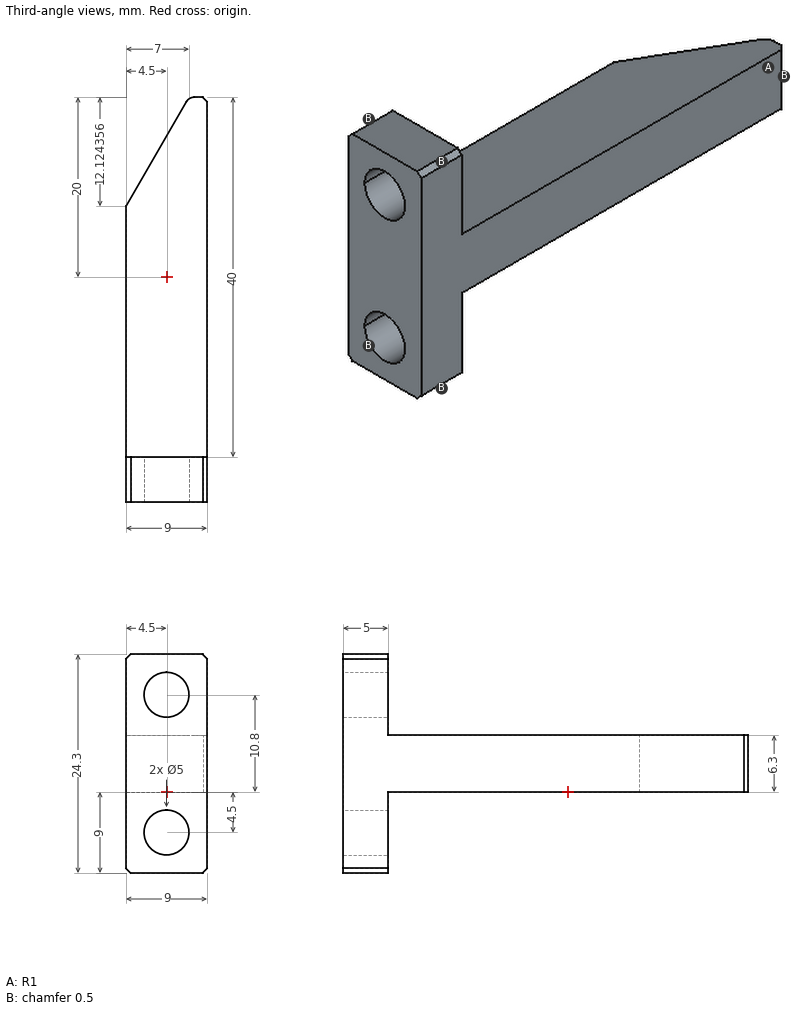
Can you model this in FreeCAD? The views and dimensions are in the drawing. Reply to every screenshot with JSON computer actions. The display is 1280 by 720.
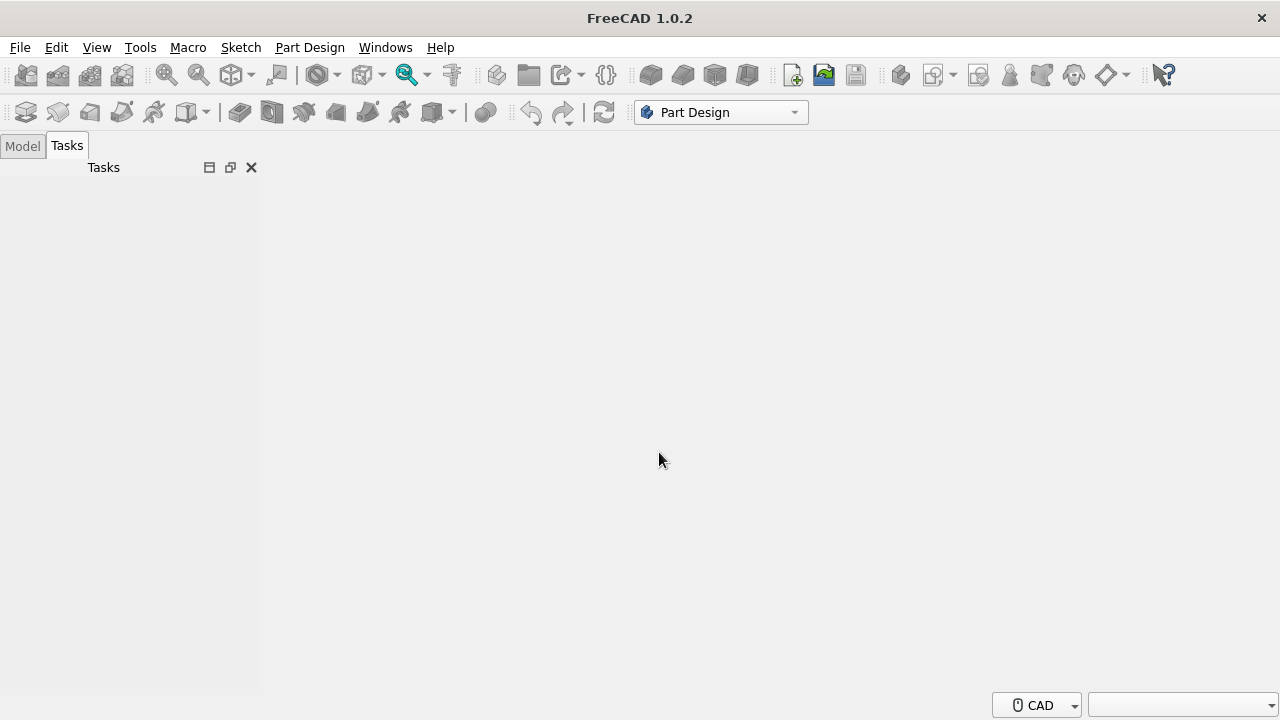
{"action": "left_click", "coordinate": [792, 76]}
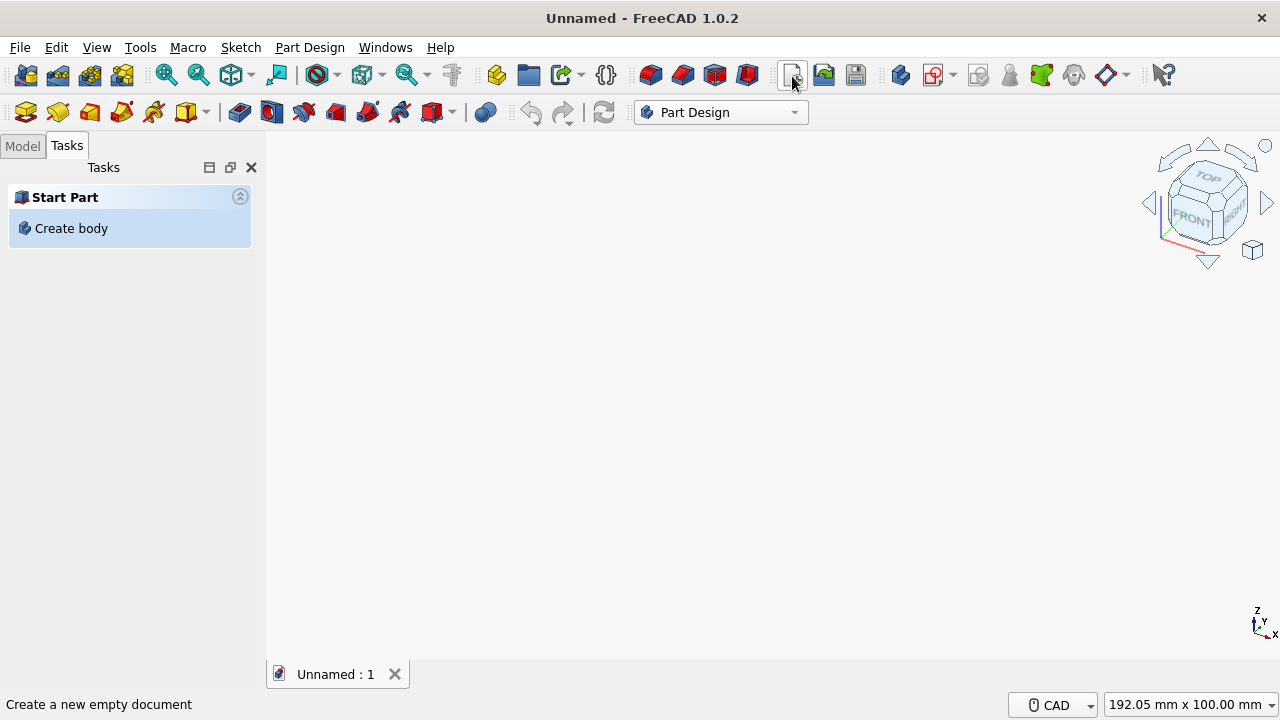
{"action": "left_click", "coordinate": [934, 76]}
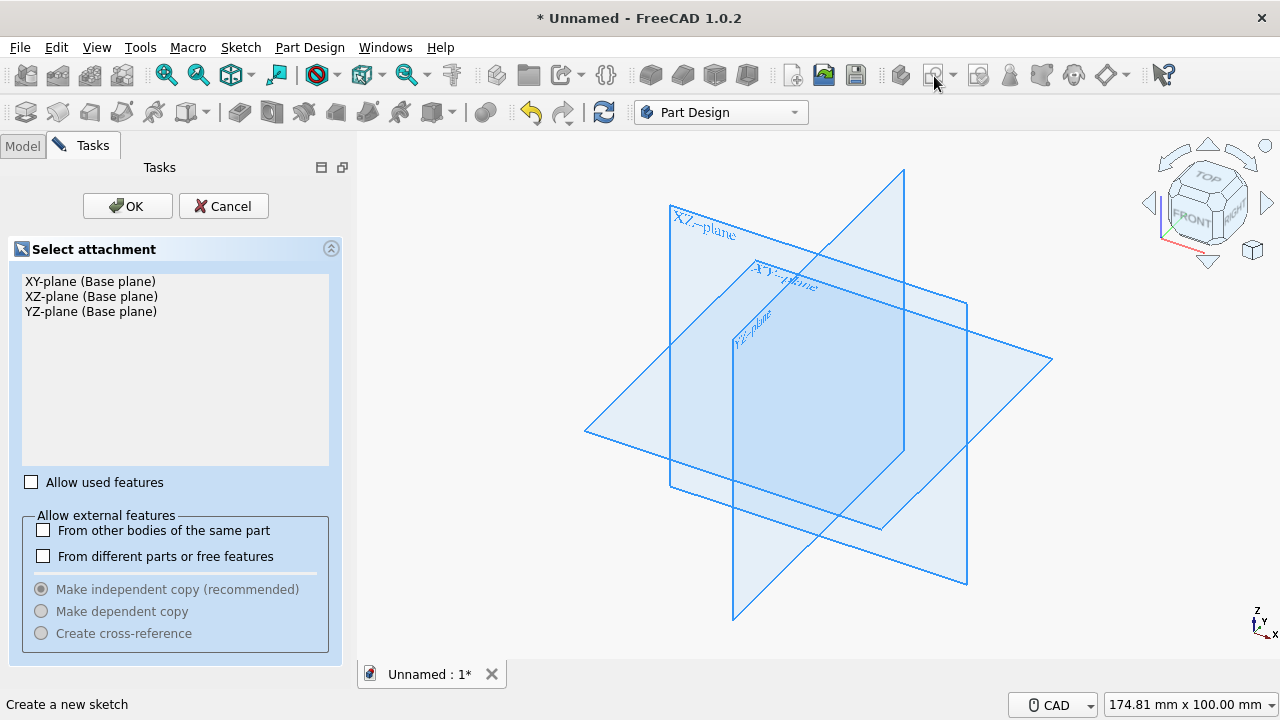
{"action": "left_click", "coordinate": [82, 282]}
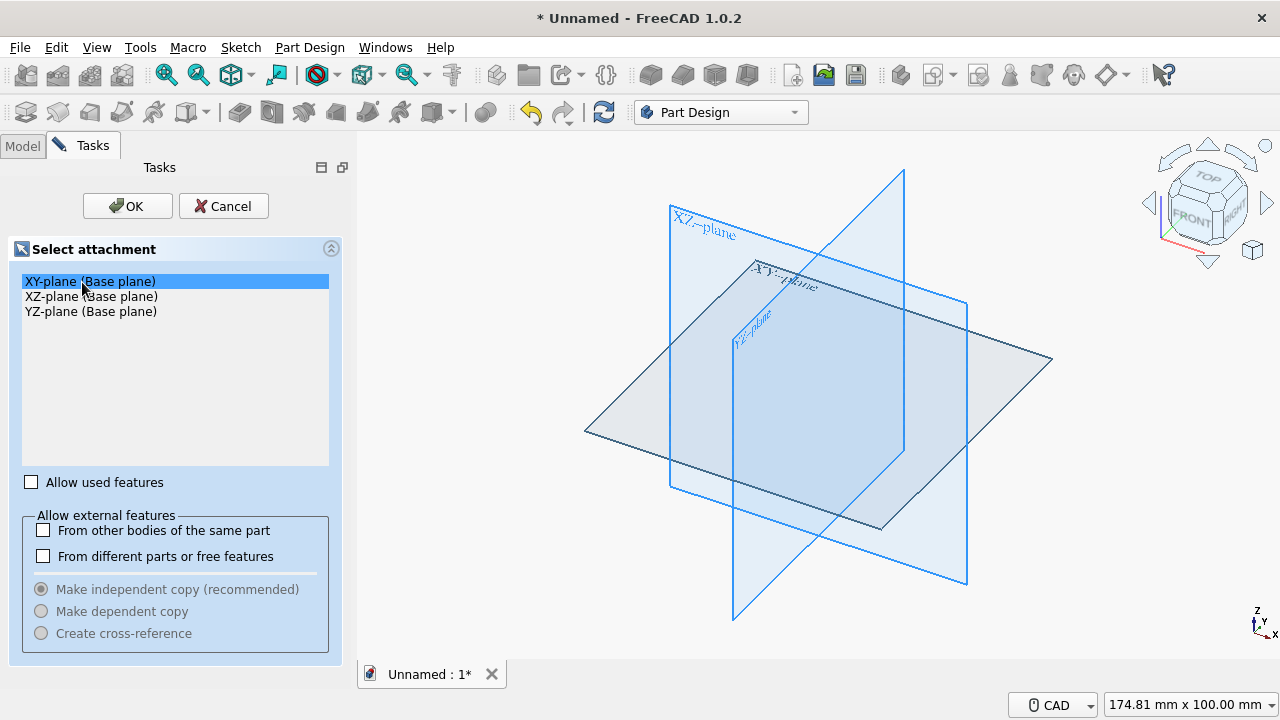
{"action": "left_click", "coordinate": [128, 206]}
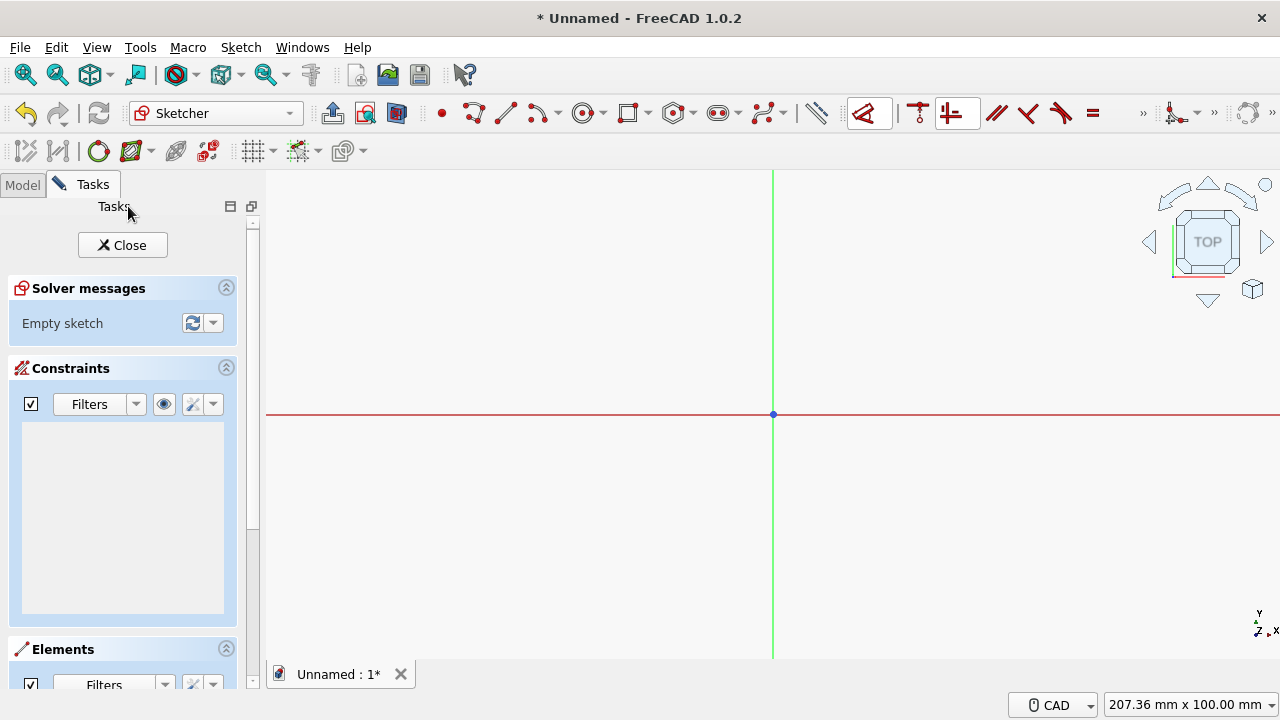
{"action": "scroll", "coordinate": [912, 414], "scroll_direction": "up", "scroll_amount": 2}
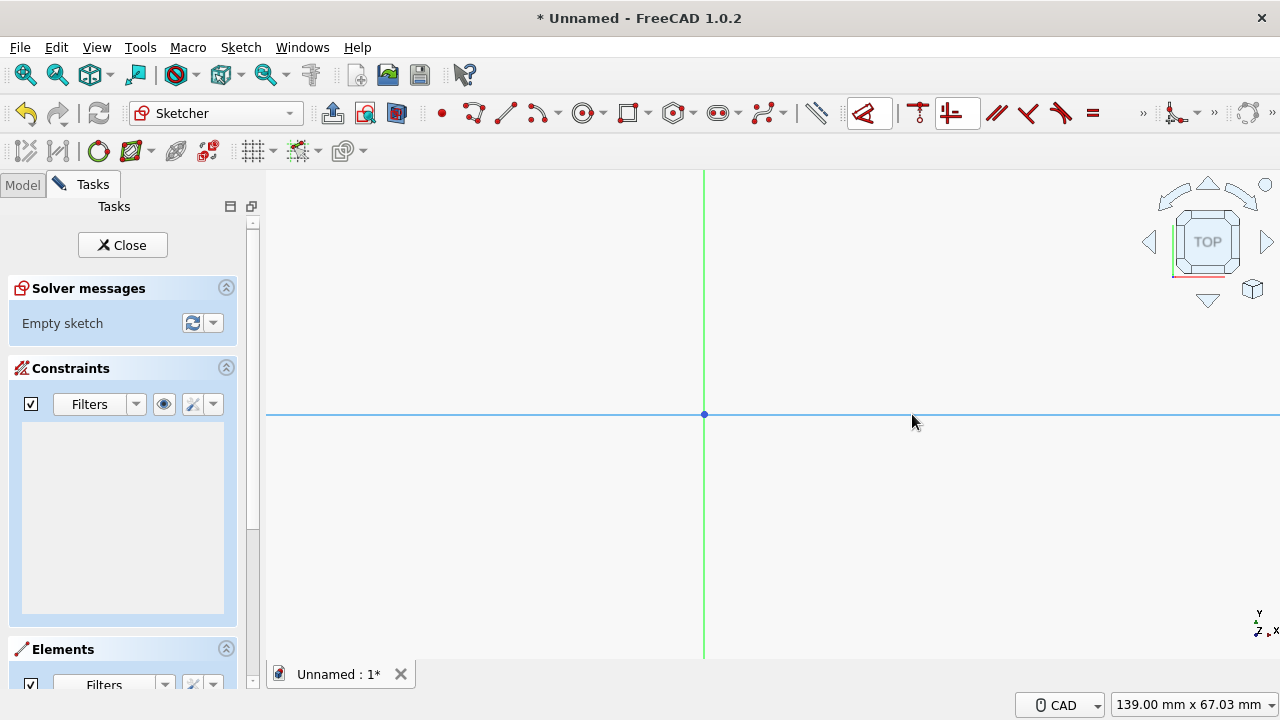
{"action": "key", "text": "g v"}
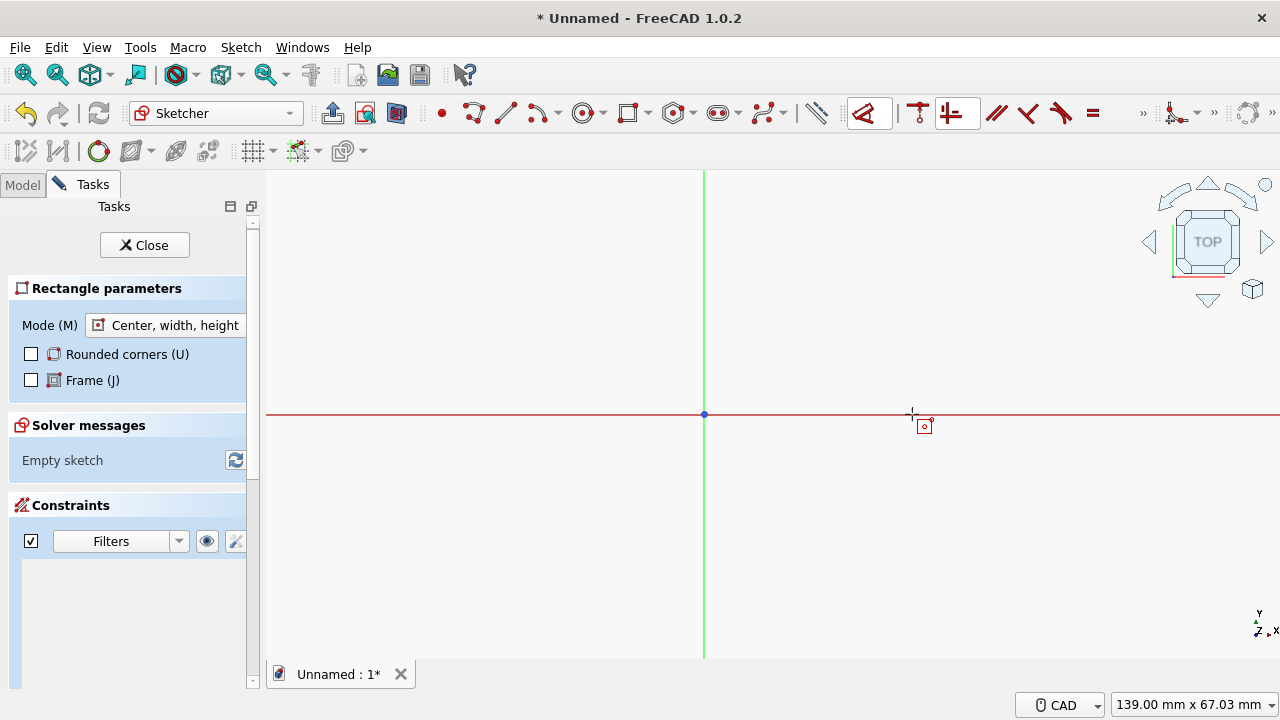
{"action": "left_click", "coordinate": [704, 414]}
{"action": "left_click", "coordinate": [737, 269]}
{"action": "key", "text": "Escape"}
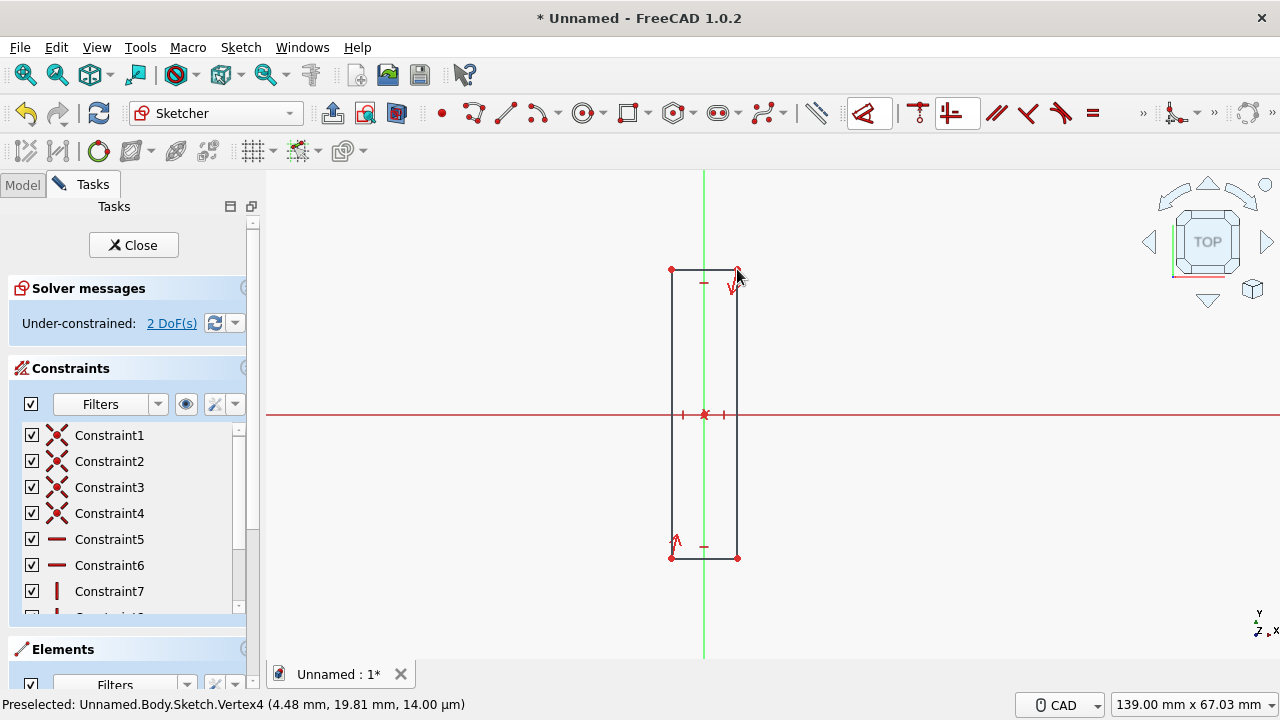
{"action": "left_click", "coordinate": [864, 114]}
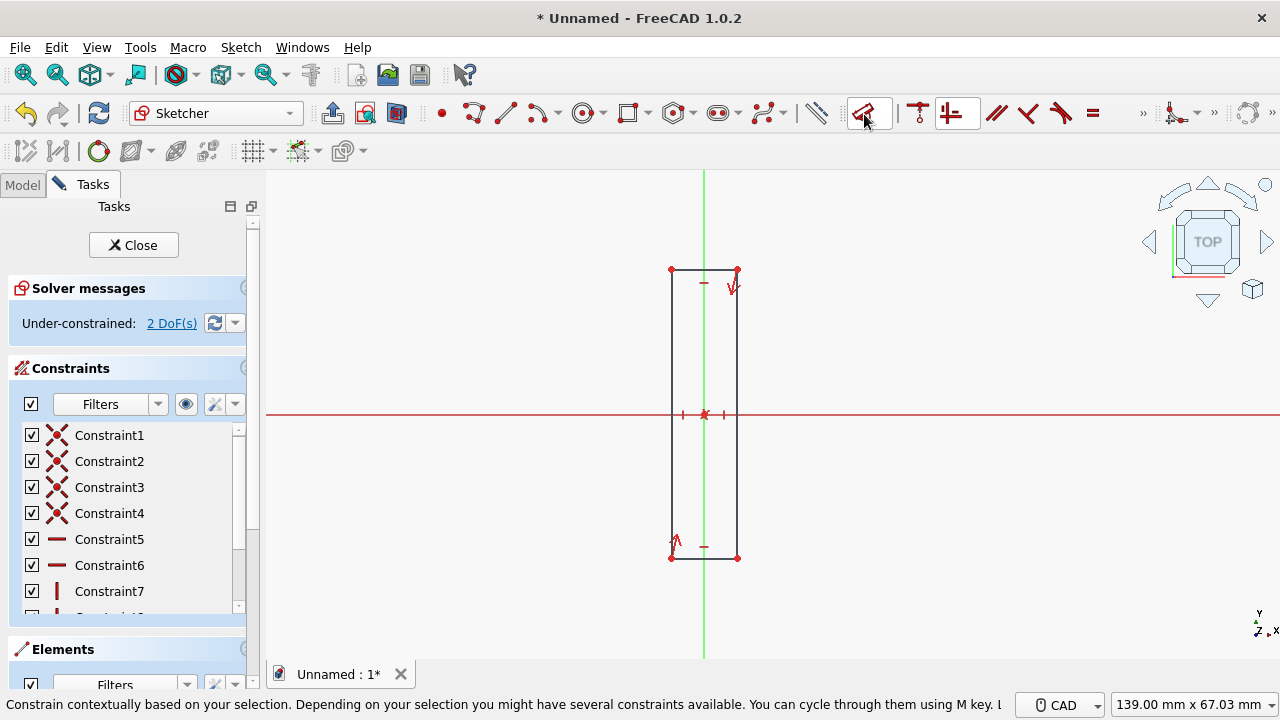
{"action": "left_click", "coordinate": [691, 559]}
{"action": "left_click", "coordinate": [689, 593]}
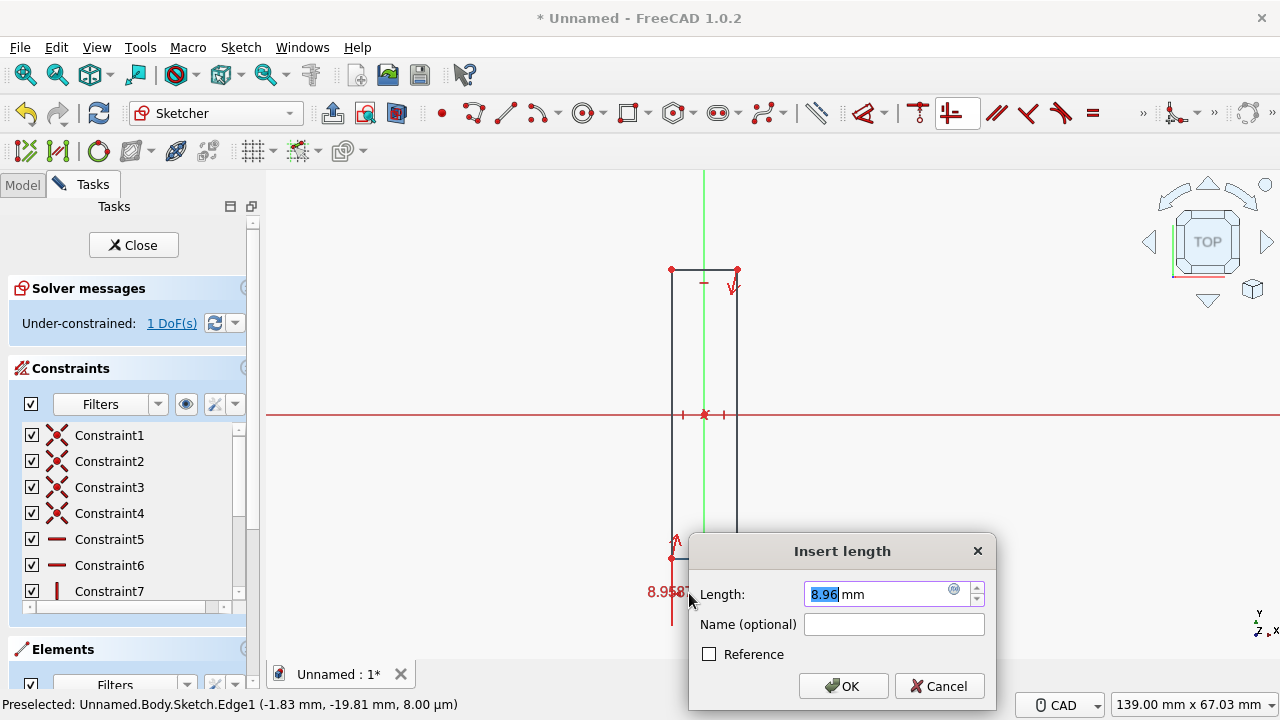
{"action": "type", "text": "9"}
{"action": "key", "text": "Return"}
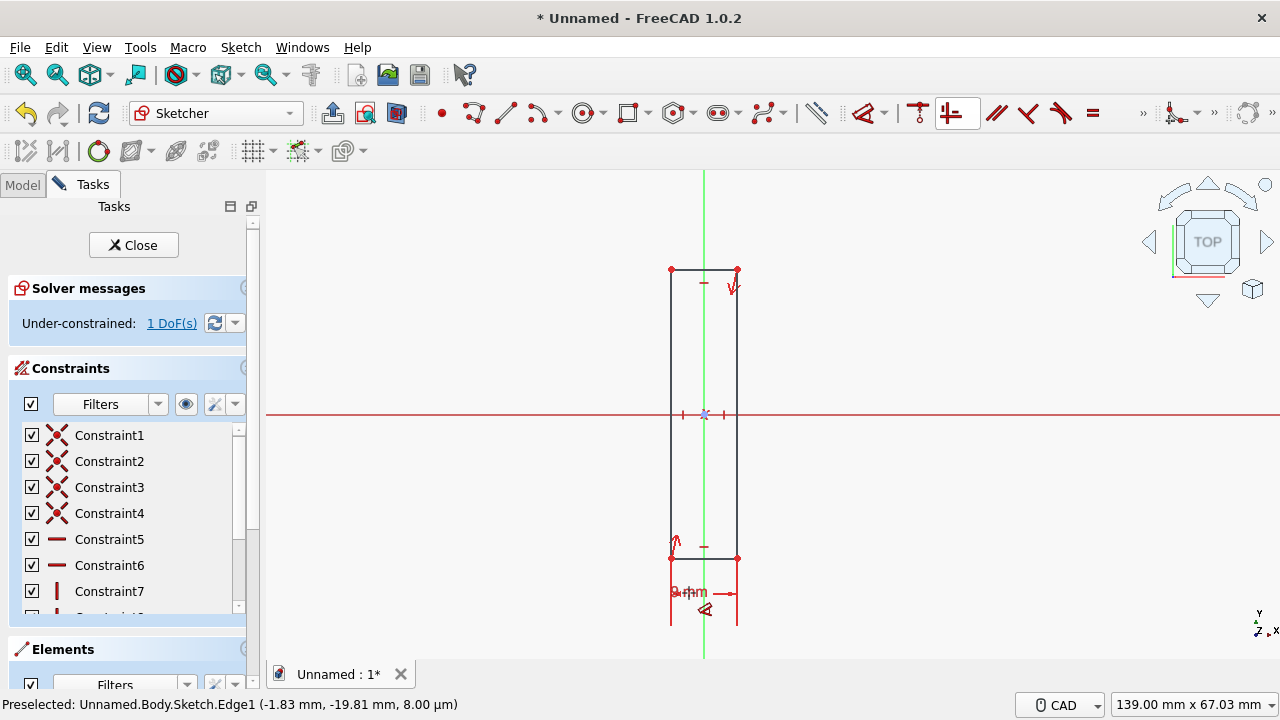
{"action": "left_click", "coordinate": [737, 472]}
{"action": "left_click", "coordinate": [771, 348]}